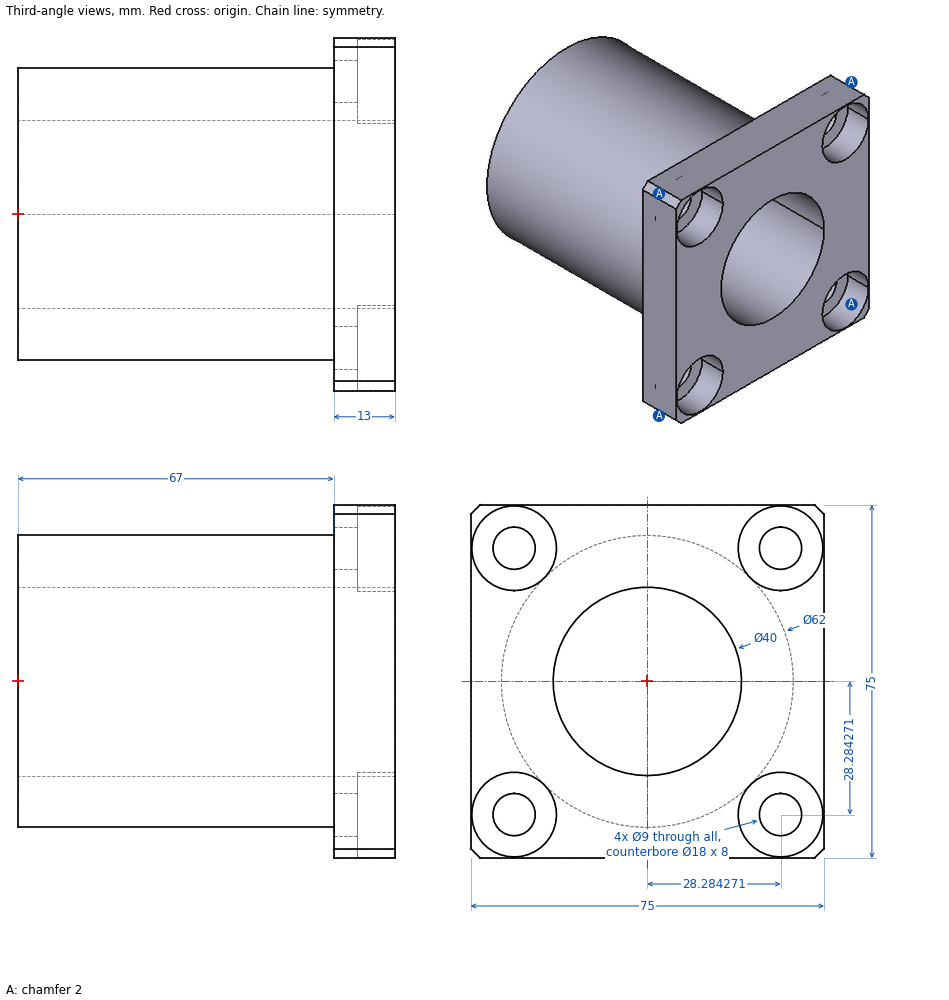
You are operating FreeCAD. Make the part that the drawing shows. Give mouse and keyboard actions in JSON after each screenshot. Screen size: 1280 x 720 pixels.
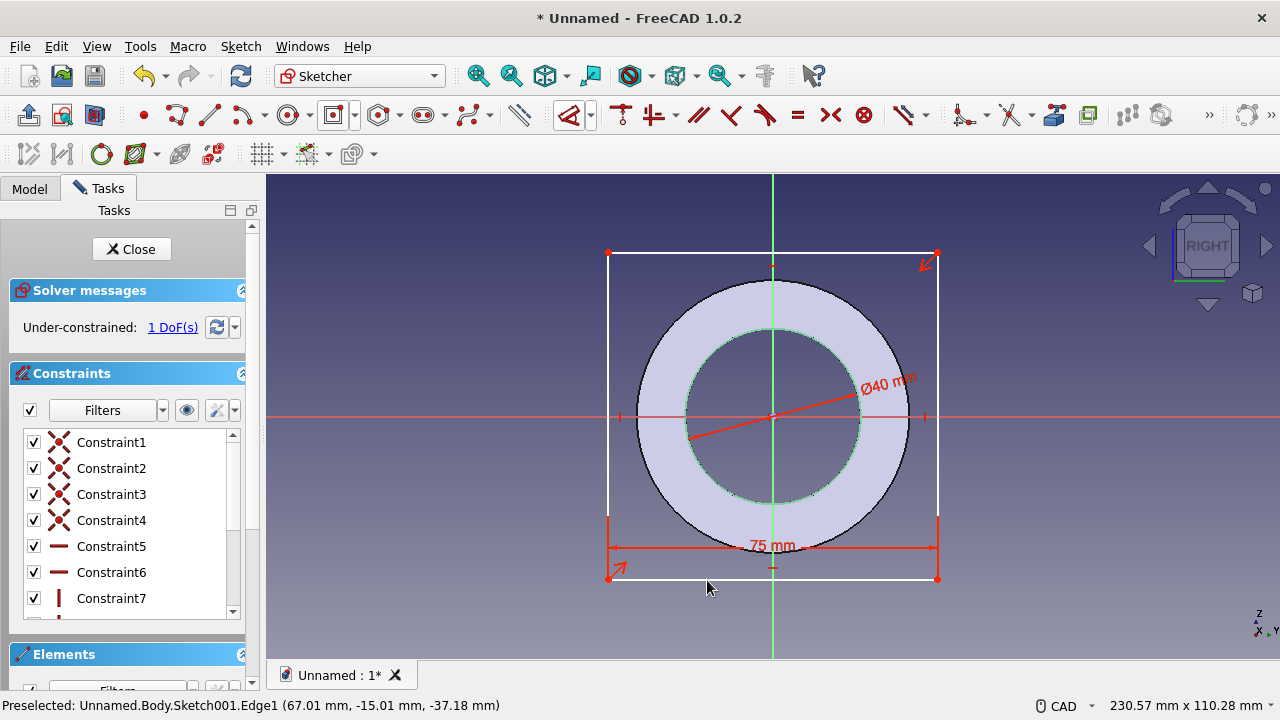
{"action": "left_click", "coordinate": [938, 482]}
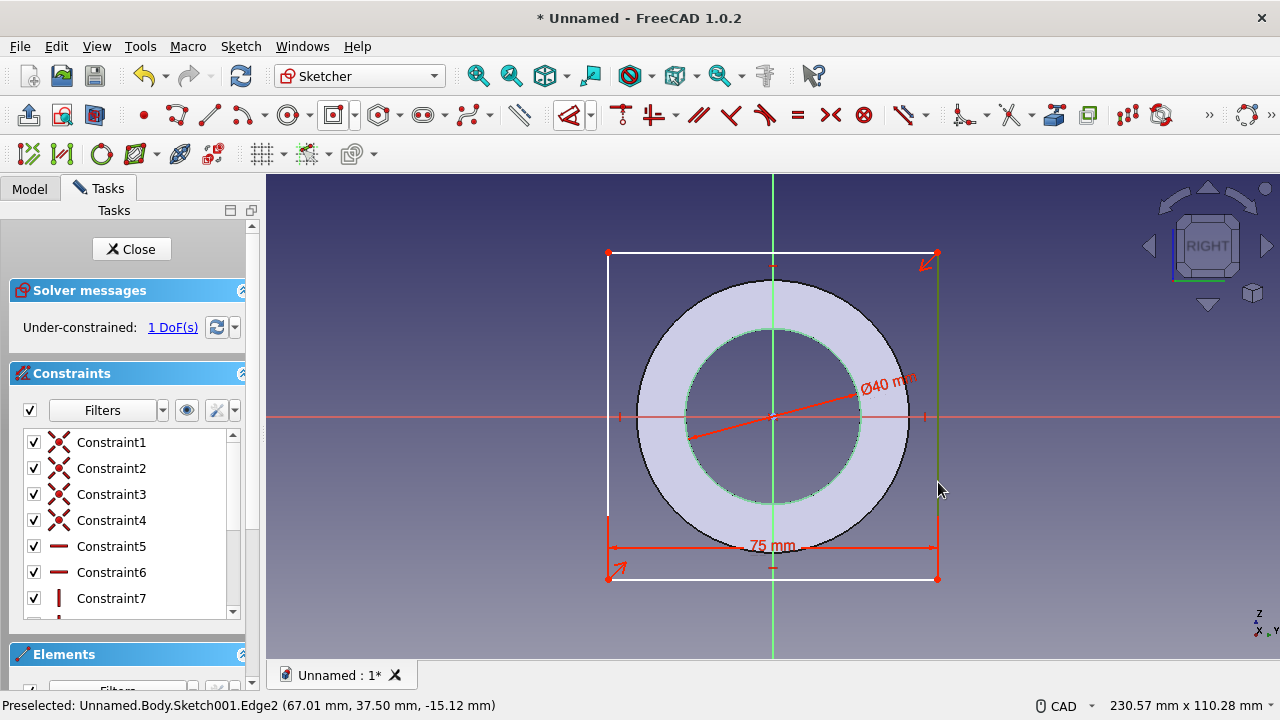
{"action": "key", "text": "i"}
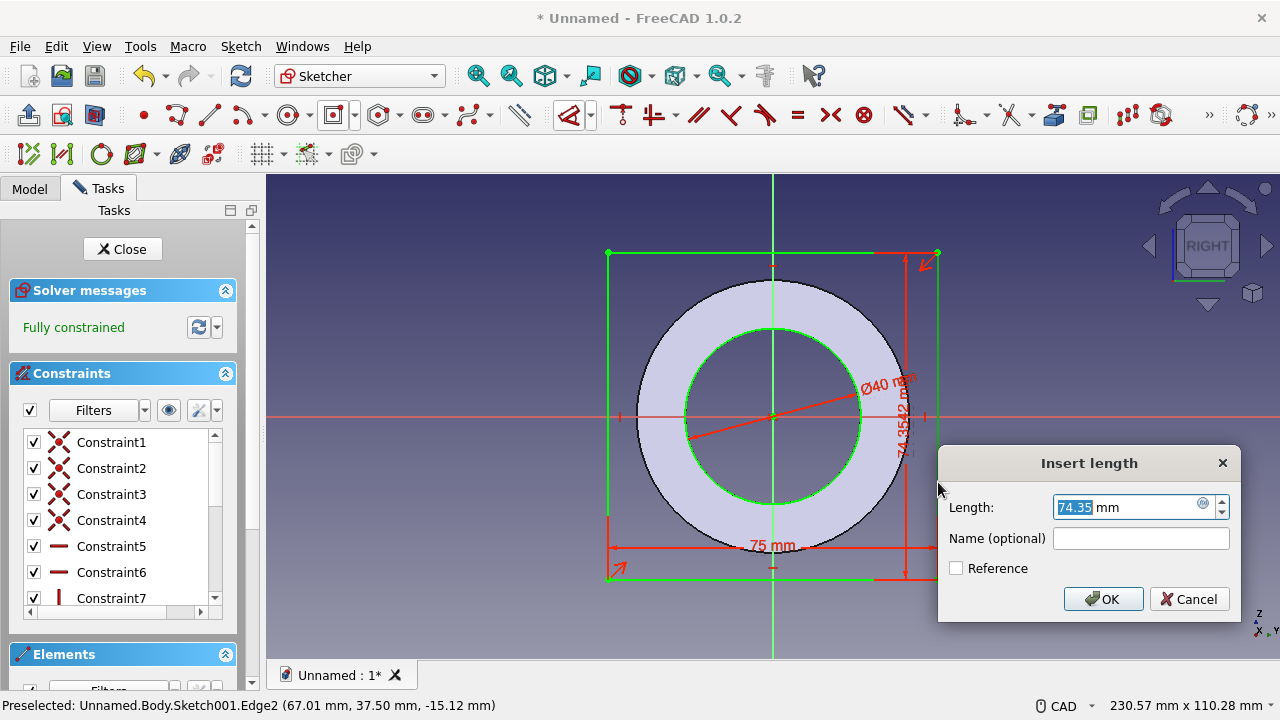
{"action": "type", "text": "75"}
{"action": "key", "text": "Return"}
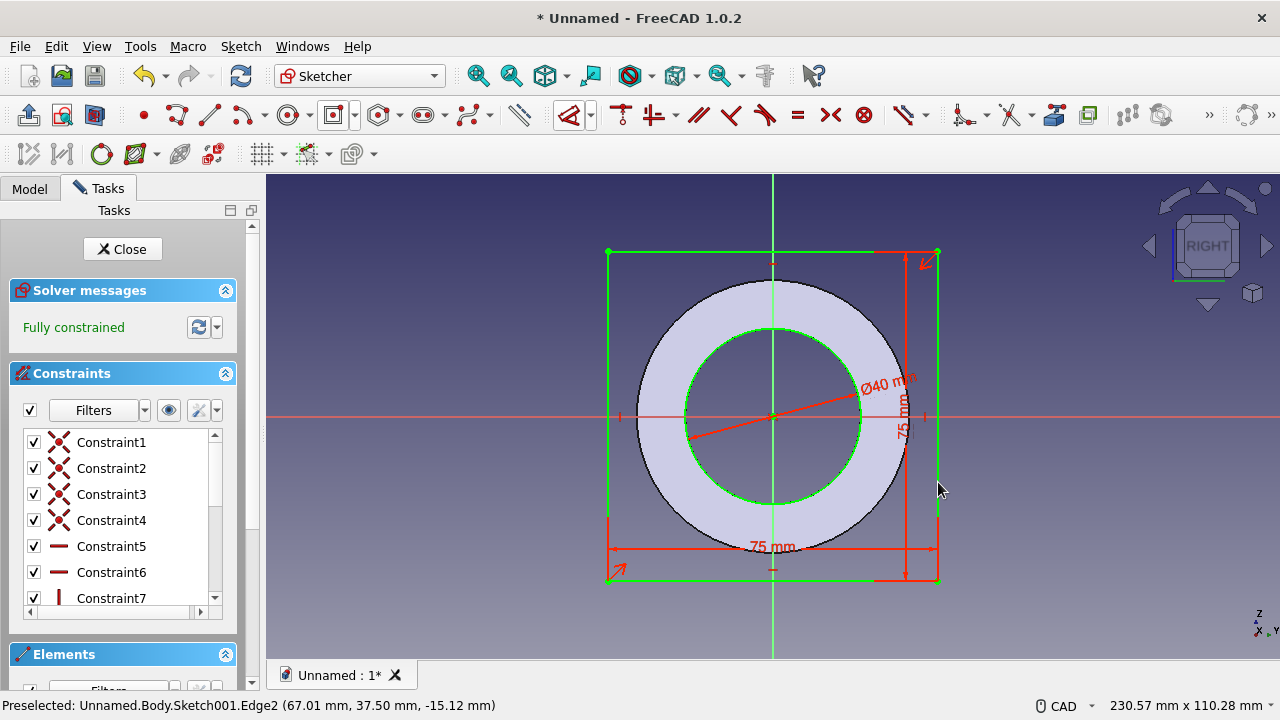
{"action": "left_click", "coordinate": [123, 249]}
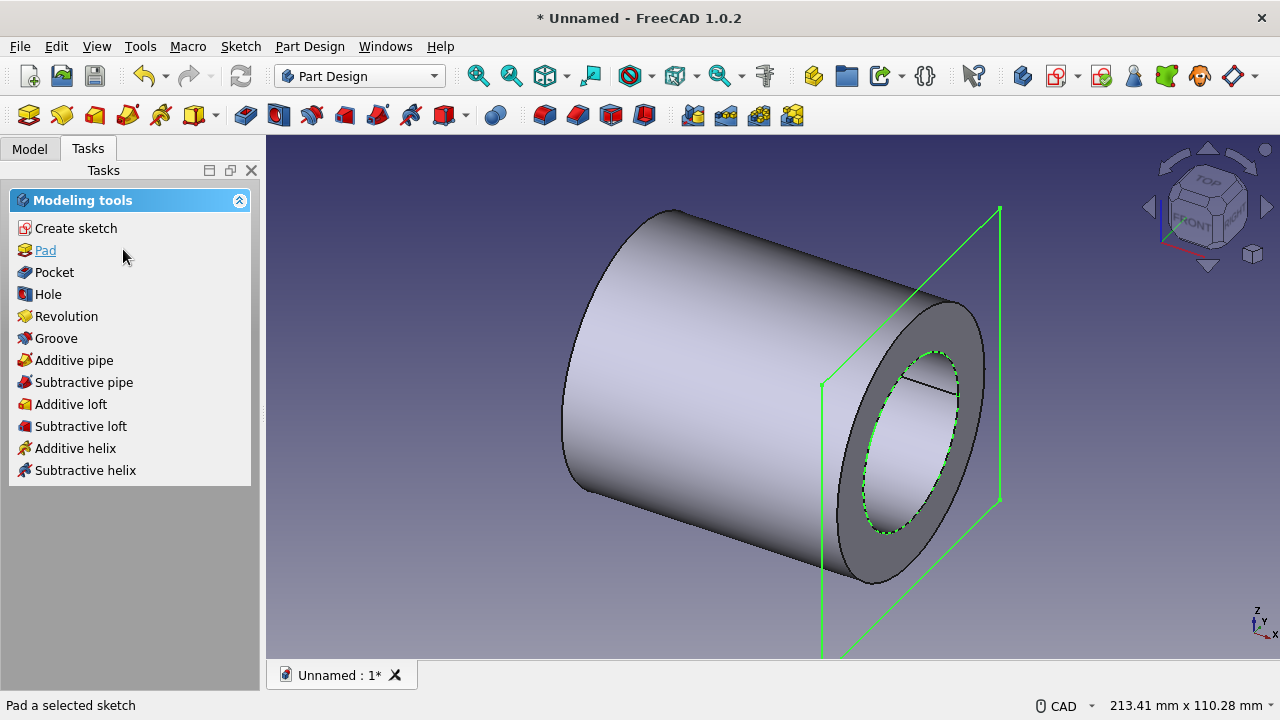
{"action": "left_click", "coordinate": [29, 116]}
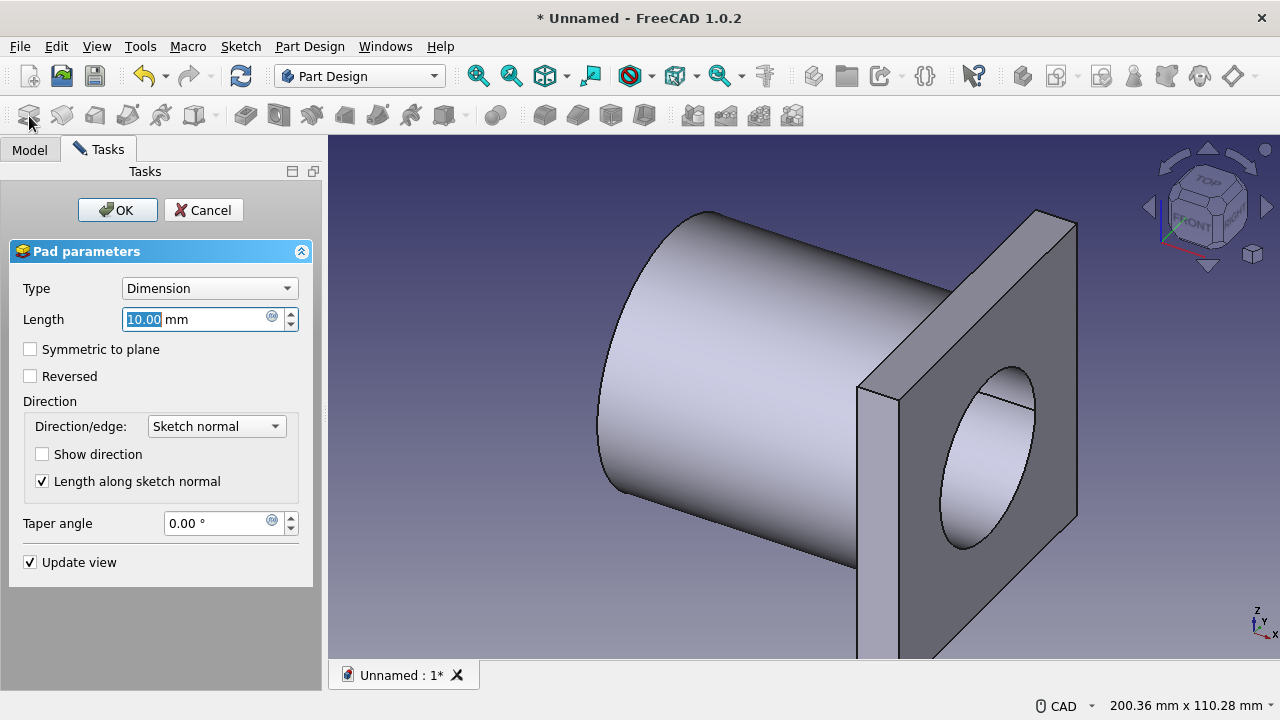
{"action": "type", "text": "13"}
{"action": "key", "text": "Tab"}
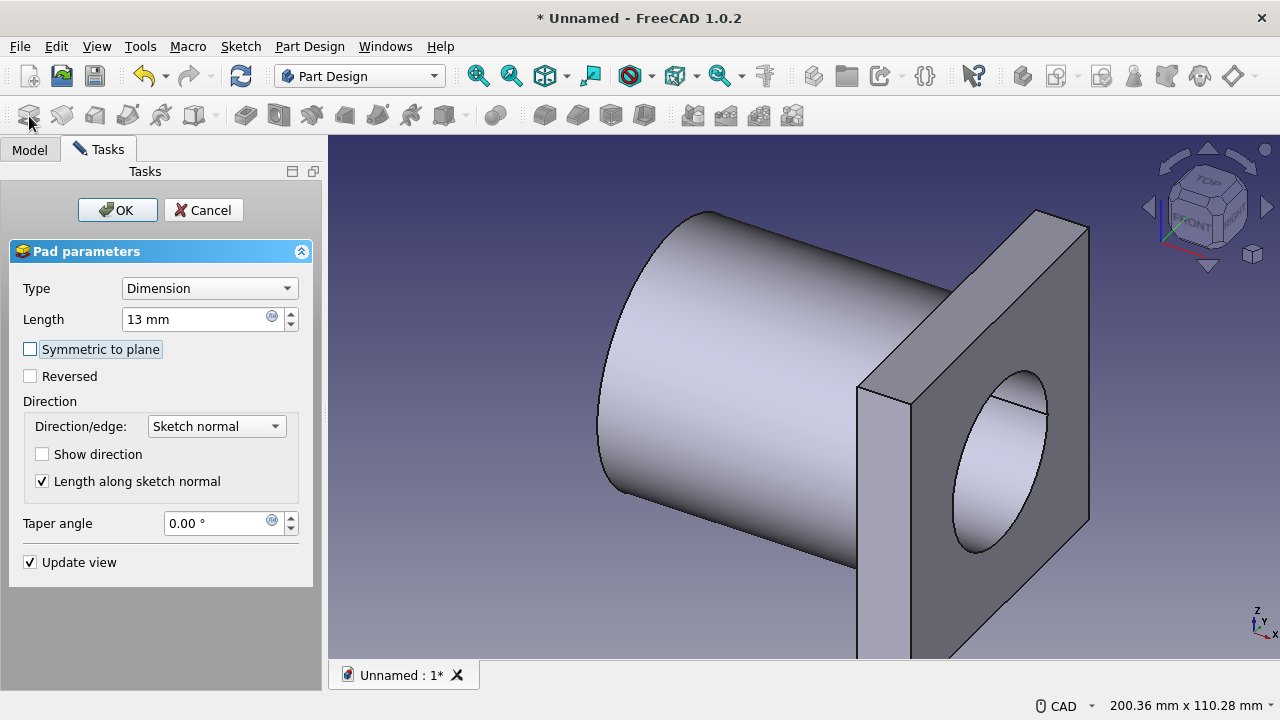
{"action": "left_click", "coordinate": [118, 210]}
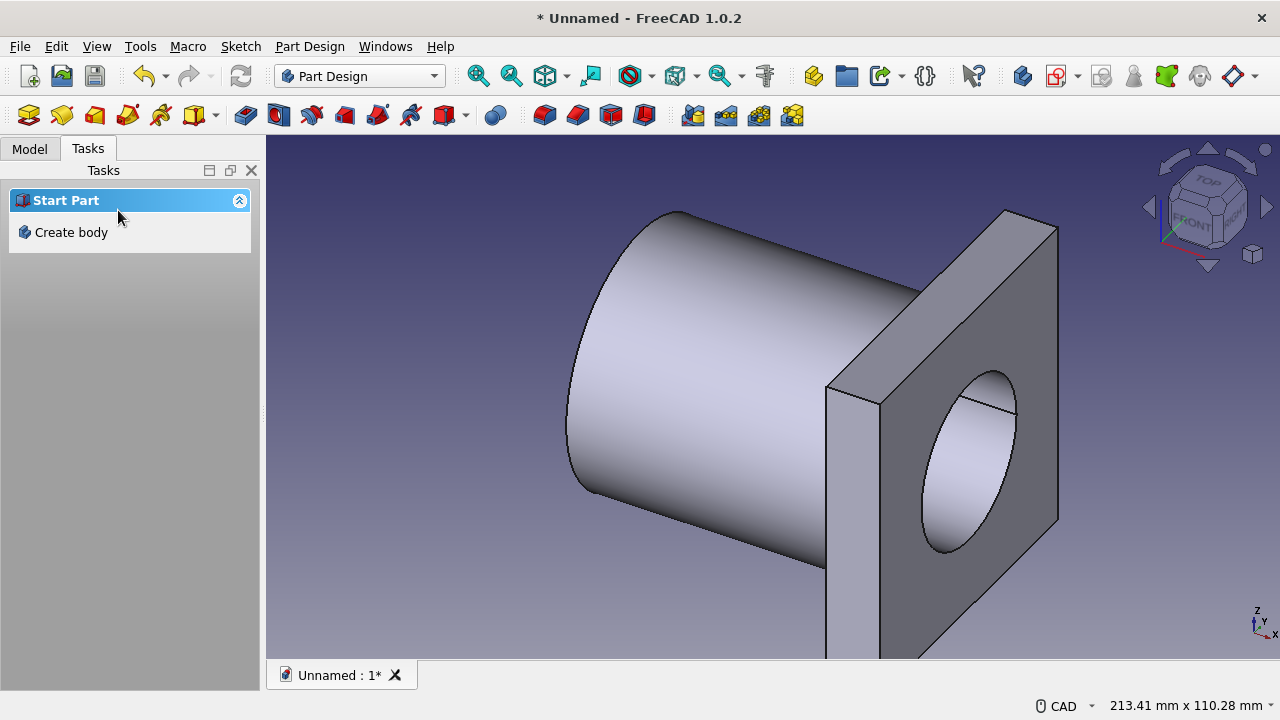
{"action": "left_click", "coordinate": [479, 76]}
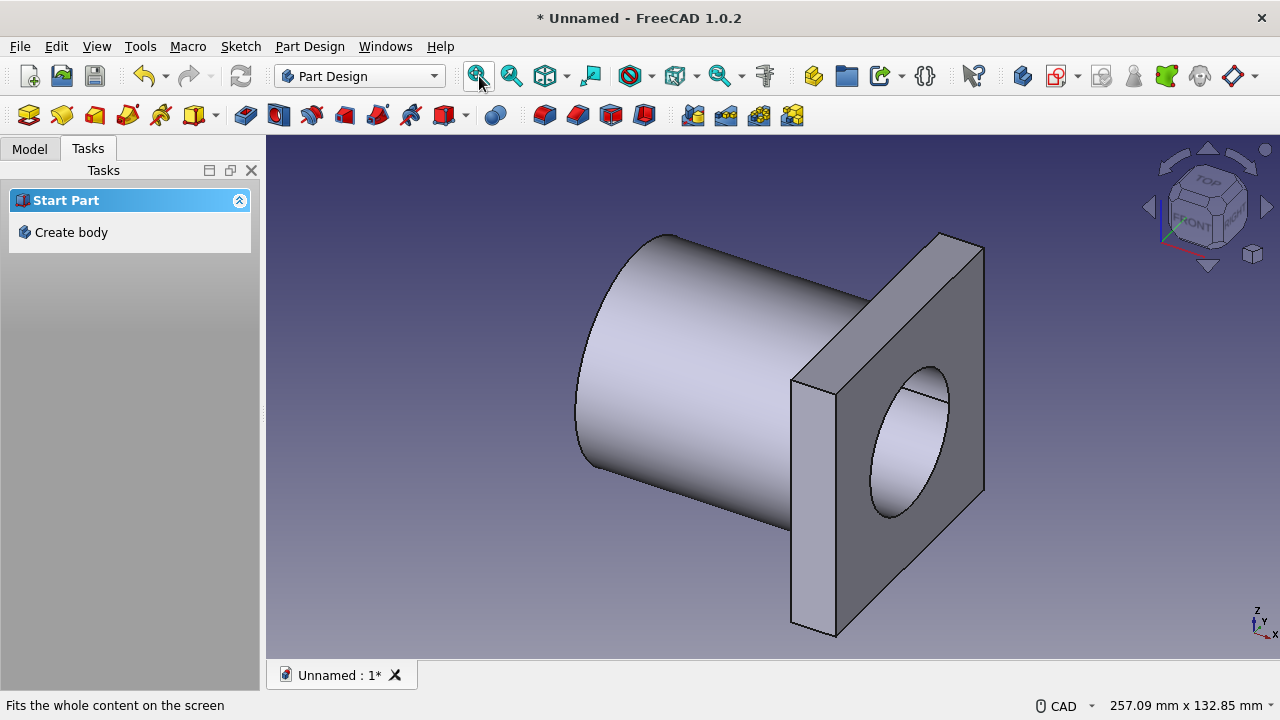
{"action": "left_click", "coordinate": [952, 330]}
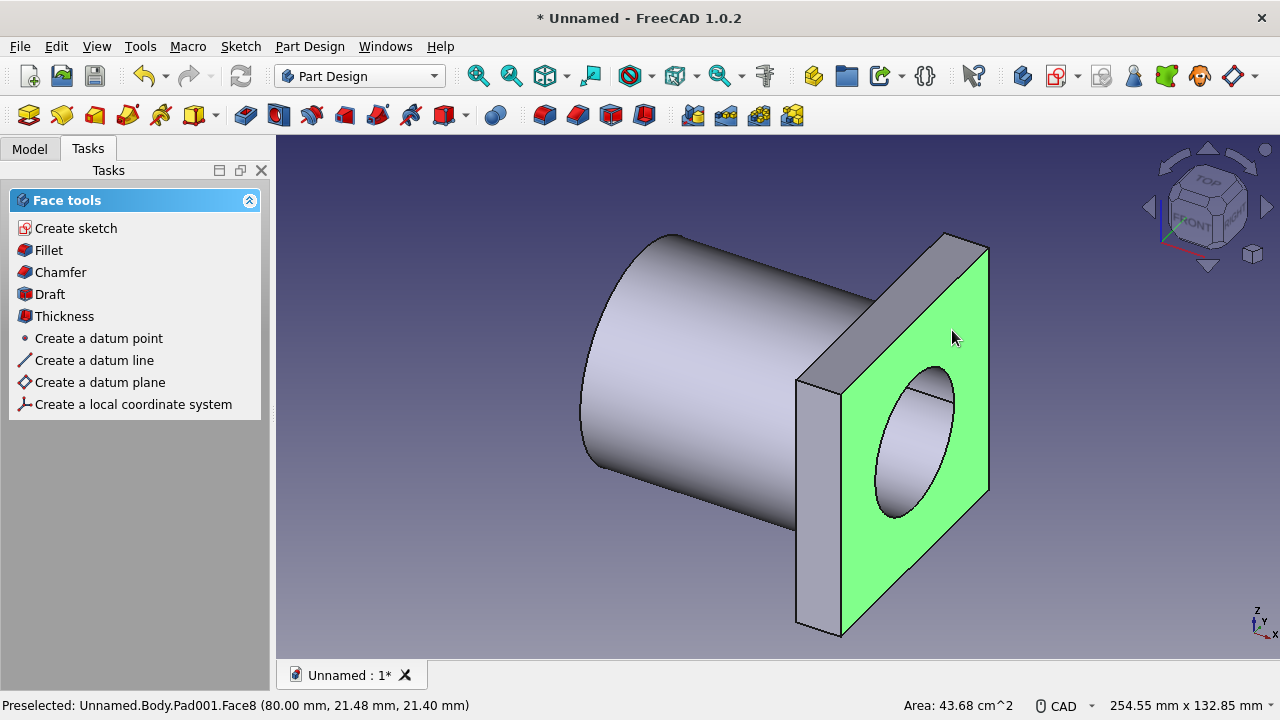
{"action": "left_click", "coordinate": [1056, 76]}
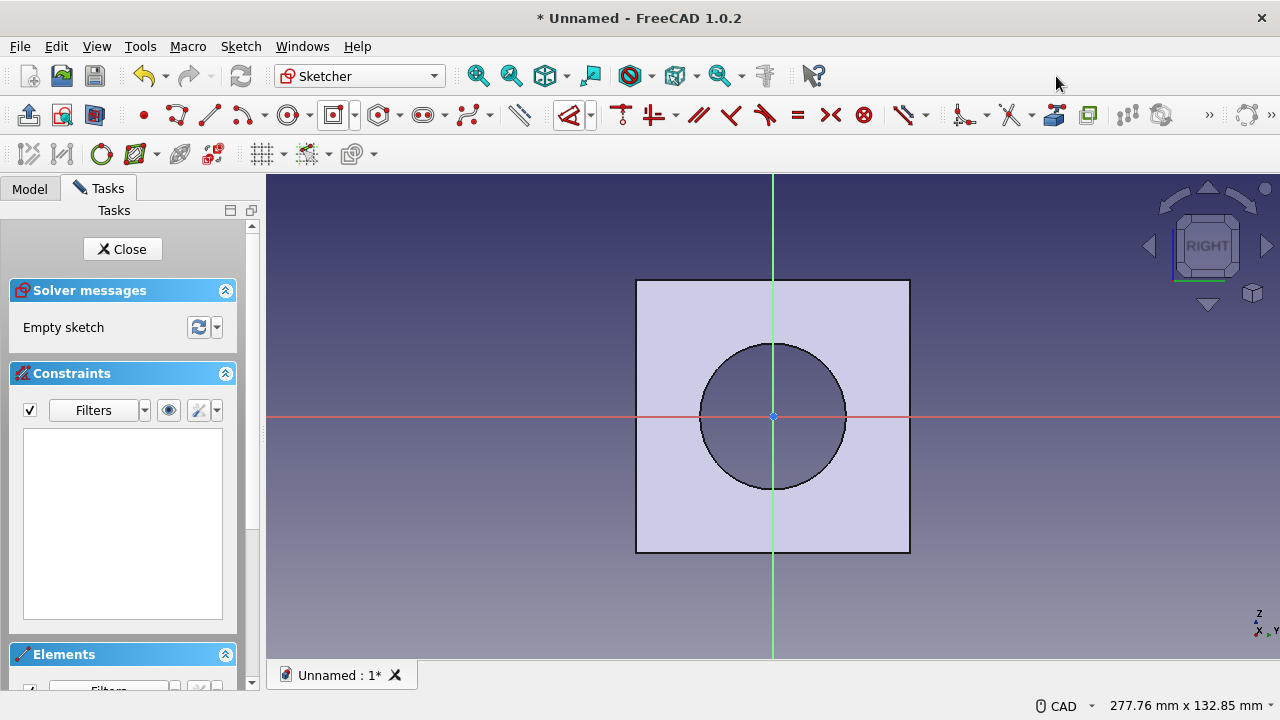
{"action": "left_click", "coordinate": [288, 116]}